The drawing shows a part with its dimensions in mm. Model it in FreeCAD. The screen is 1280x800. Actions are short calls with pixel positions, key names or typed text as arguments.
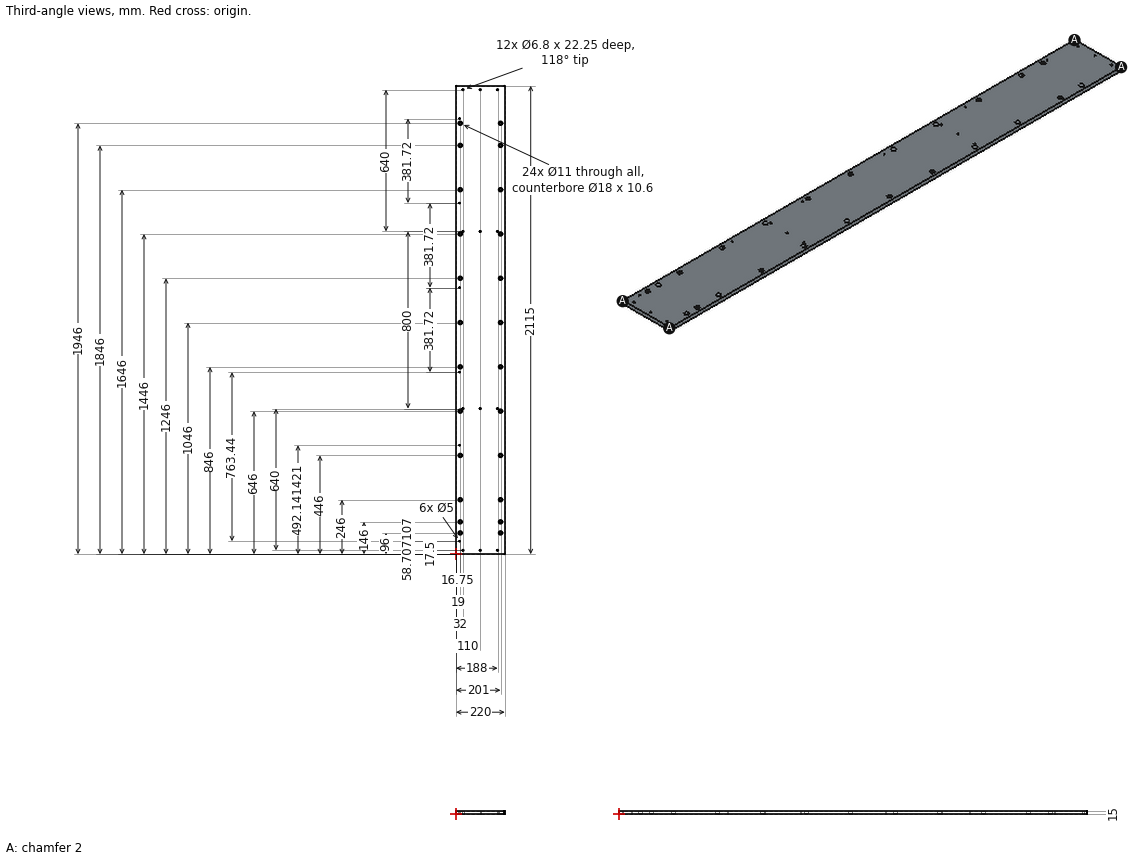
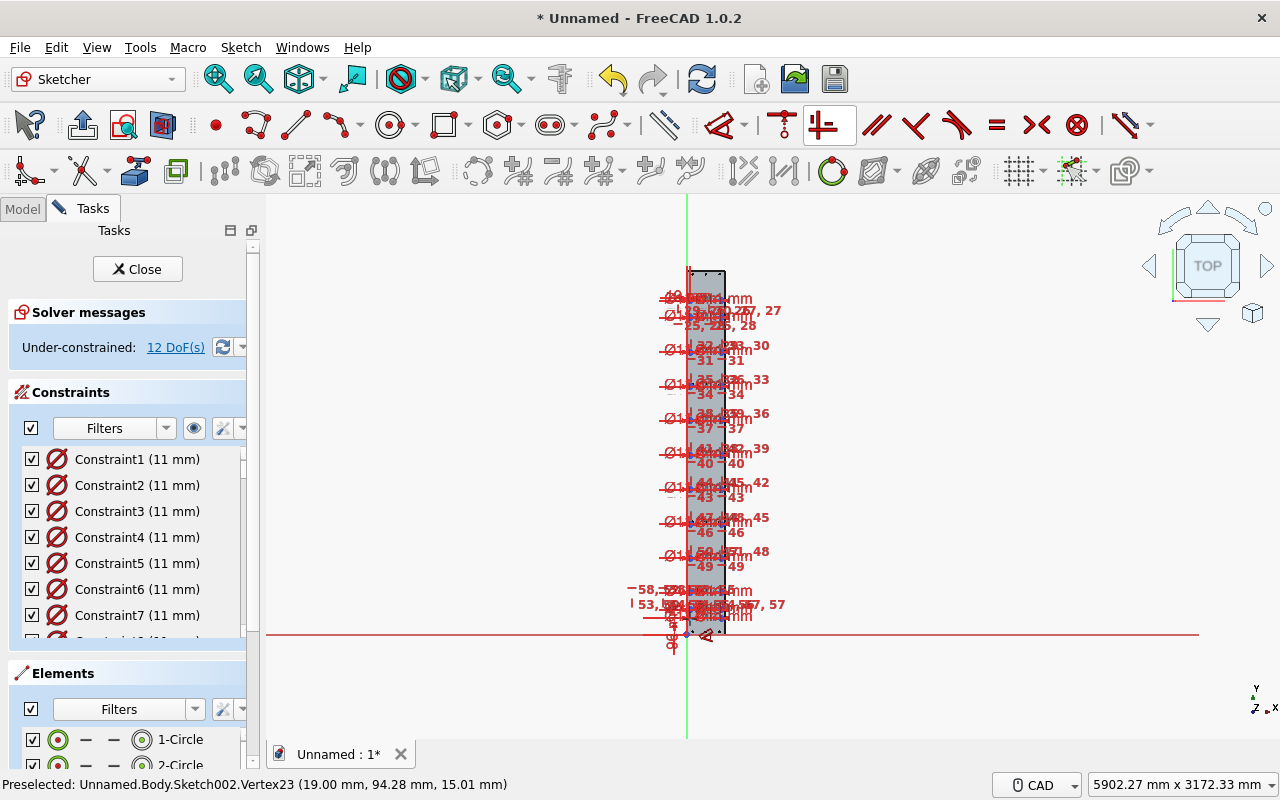
click(721, 301)
click(704, 669)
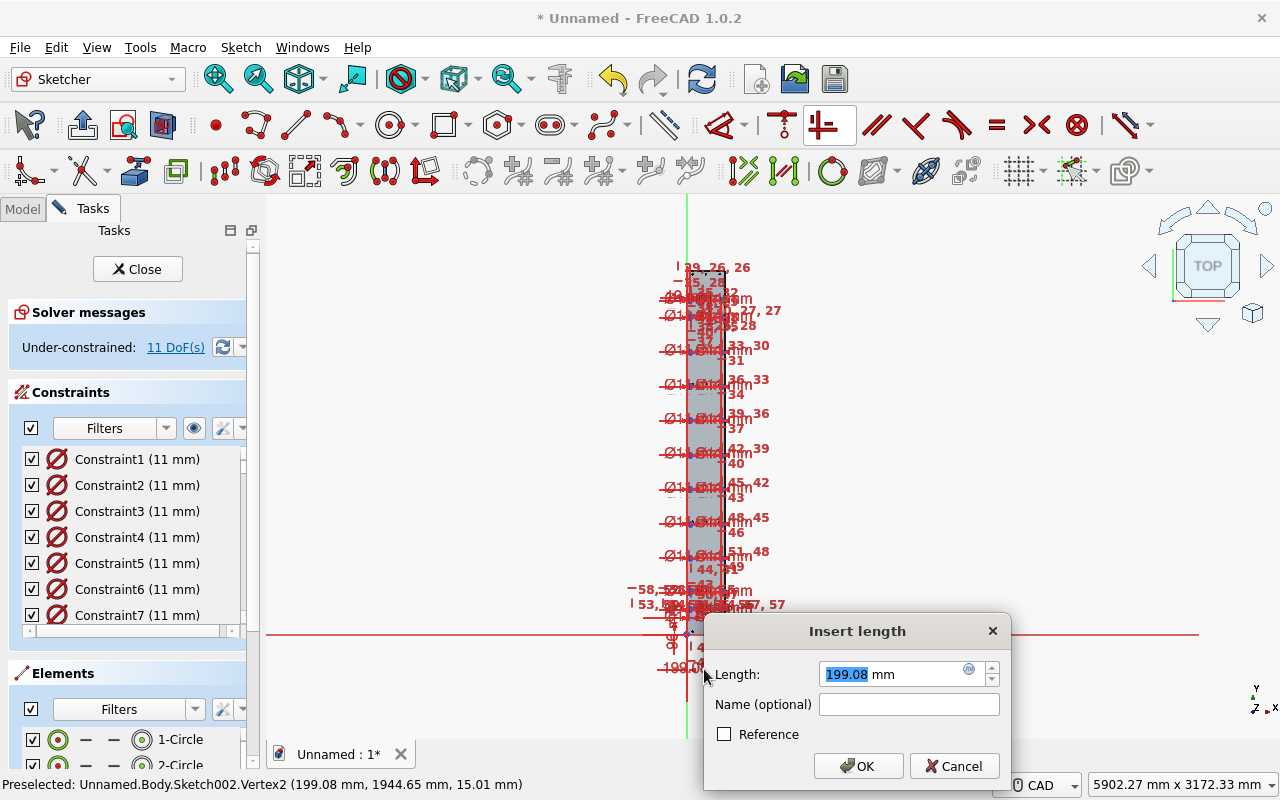
text(201)
key(Return)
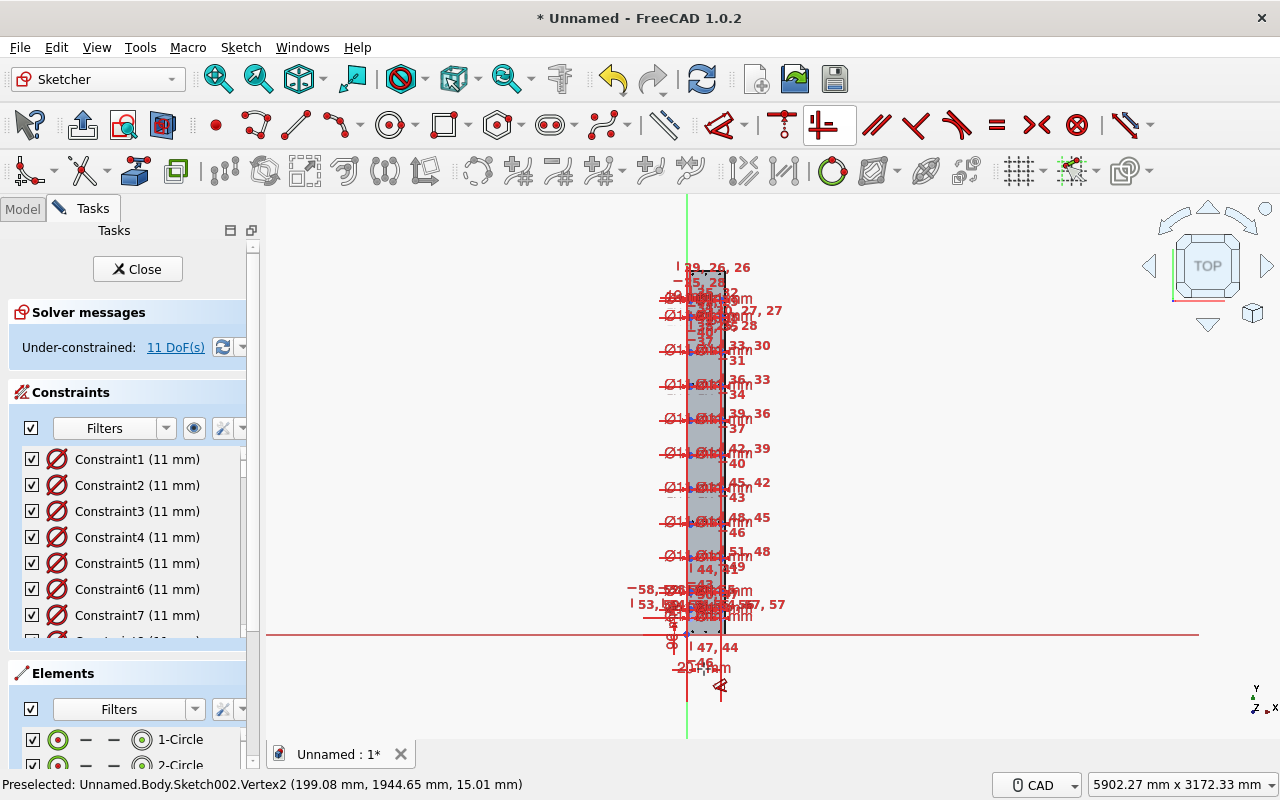
click(690, 490)
click(653, 562)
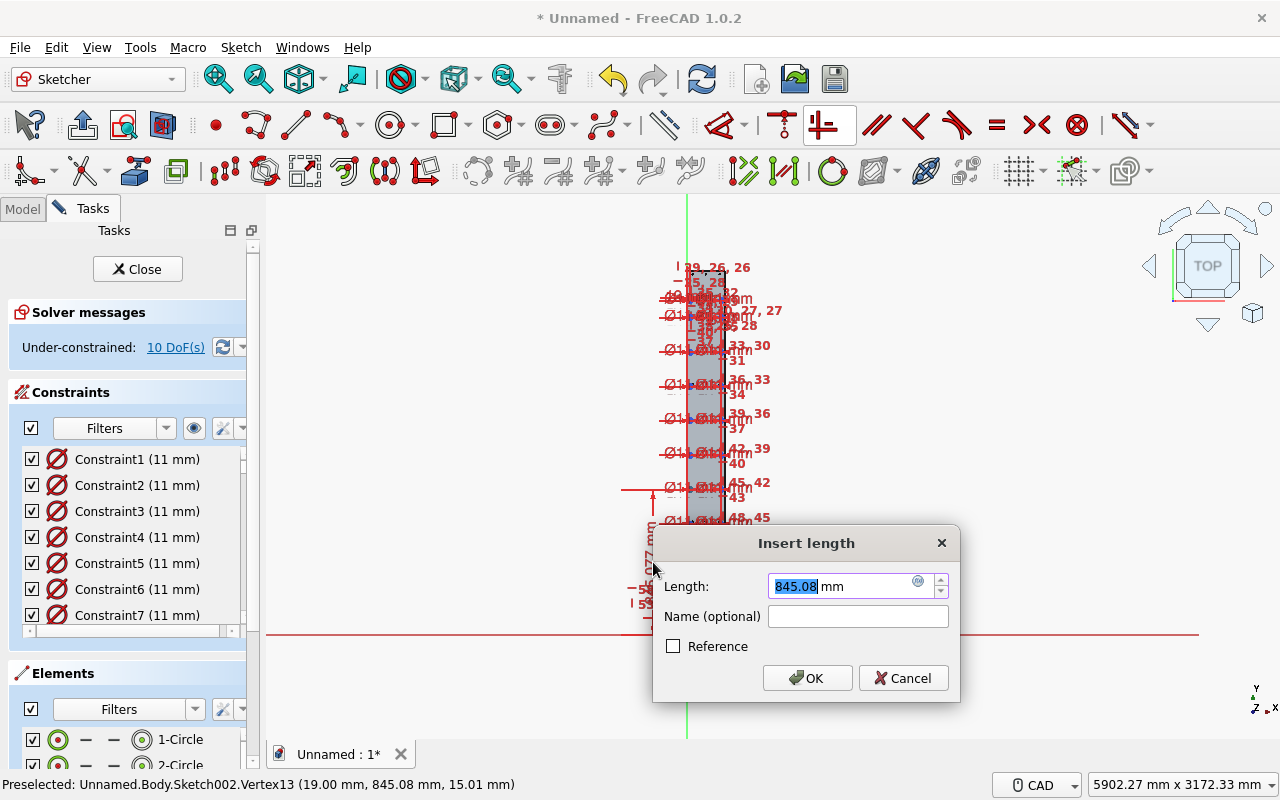
text(846)
key(Return)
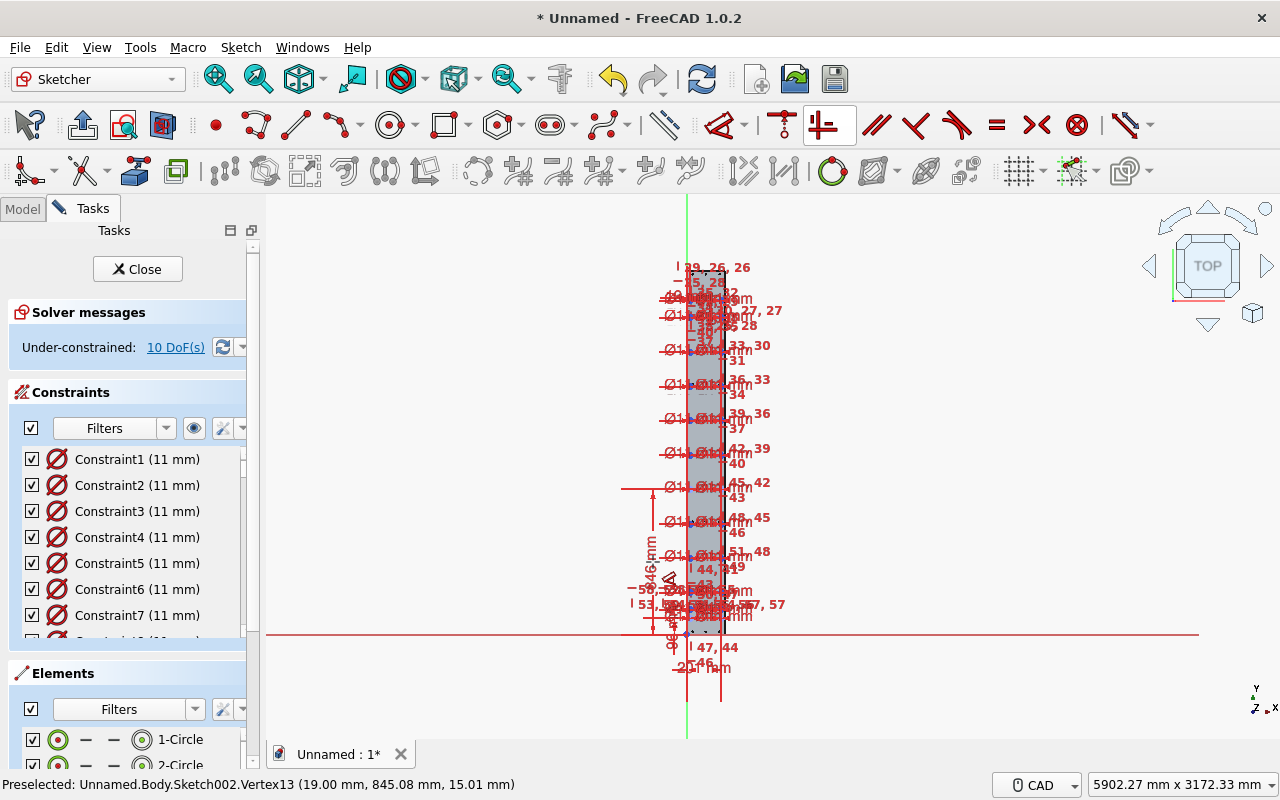
click(690, 524)
click(653, 605)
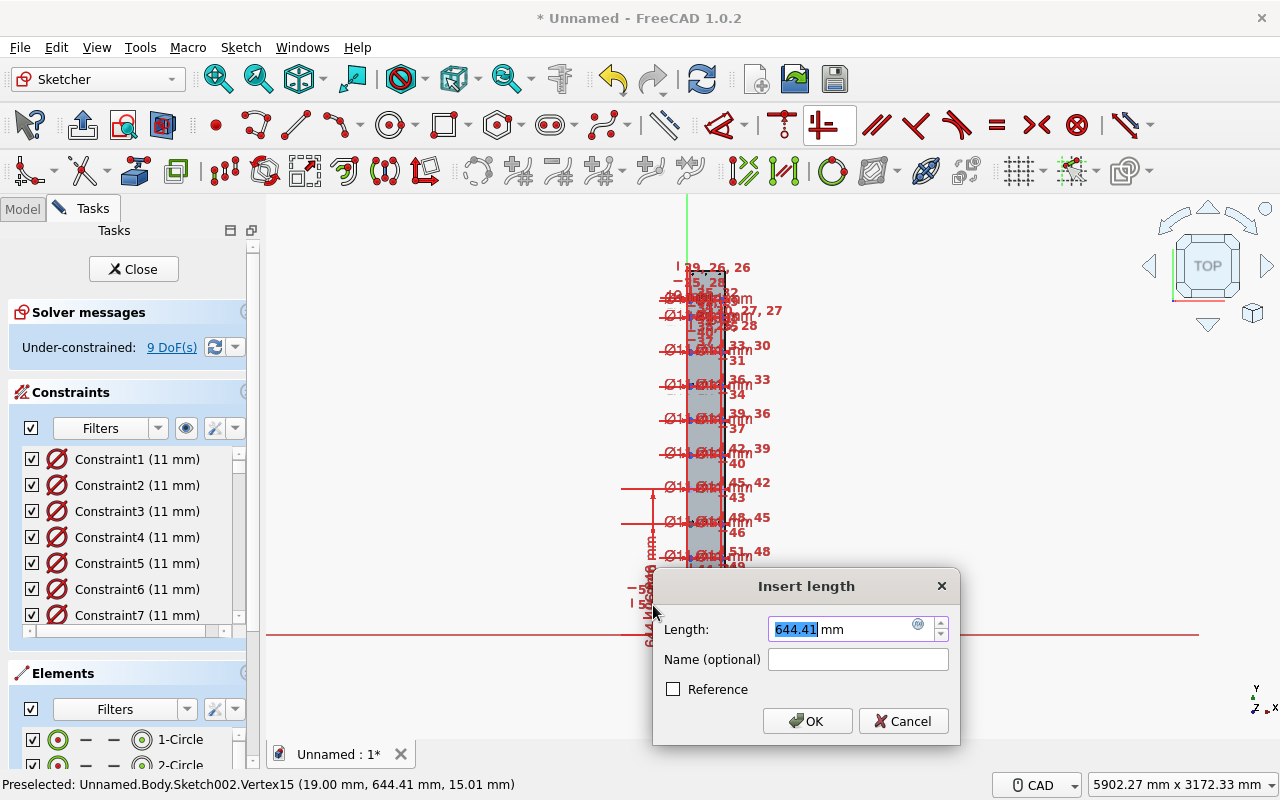
text(646)
key(Return)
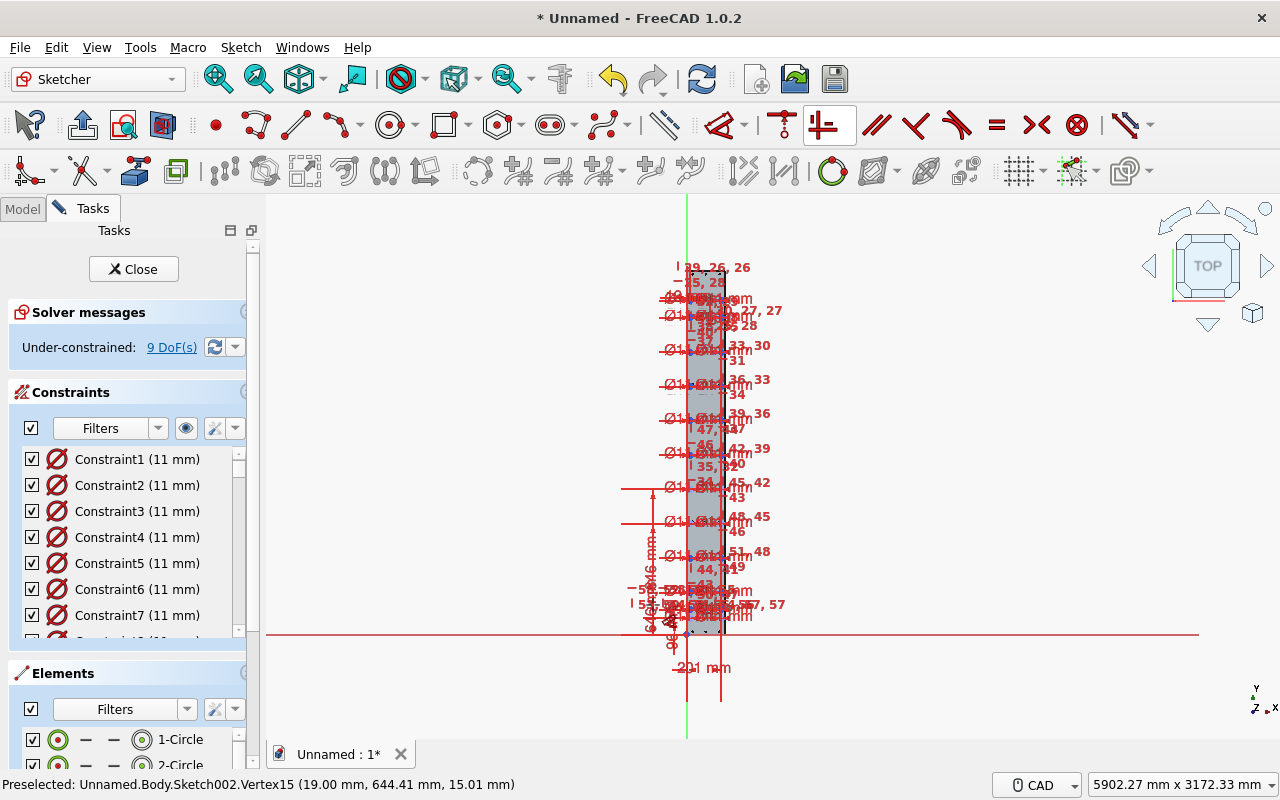
click(690, 558)
click(724, 579)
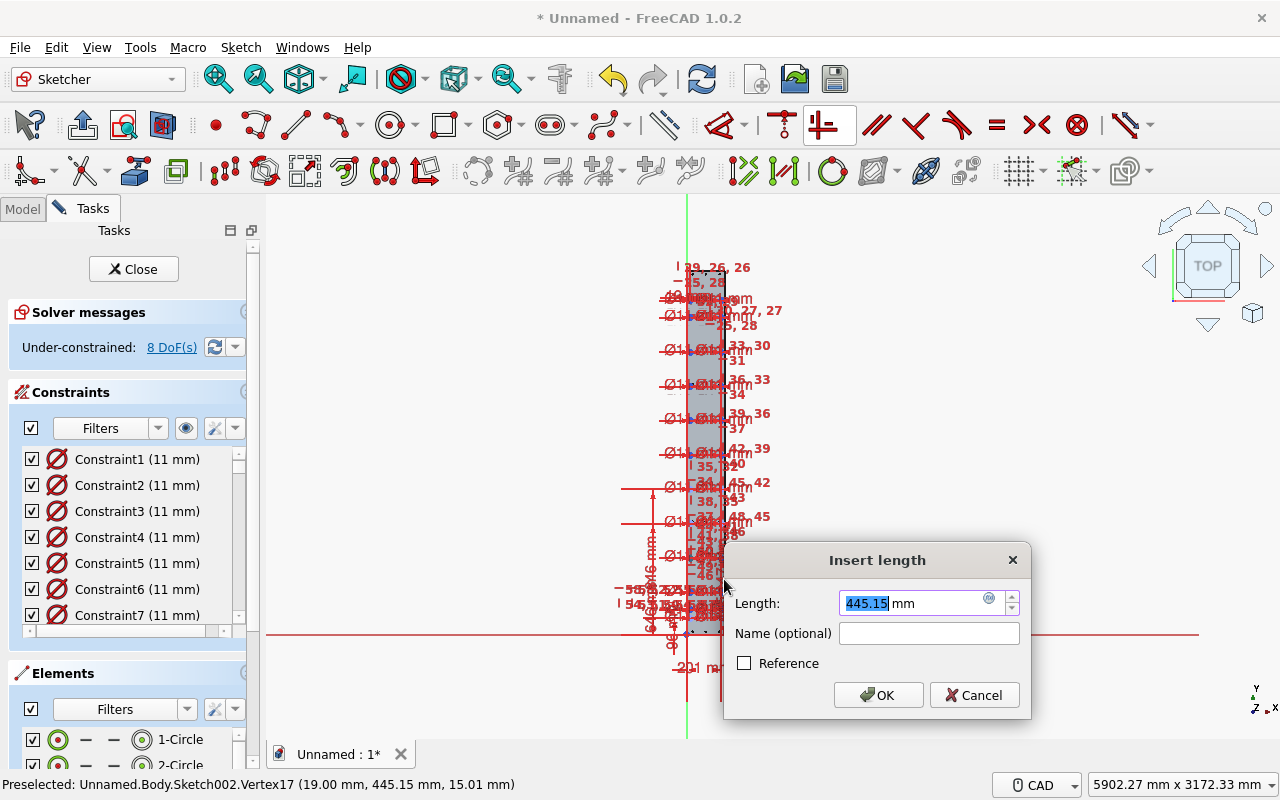
text(446)
key(Return)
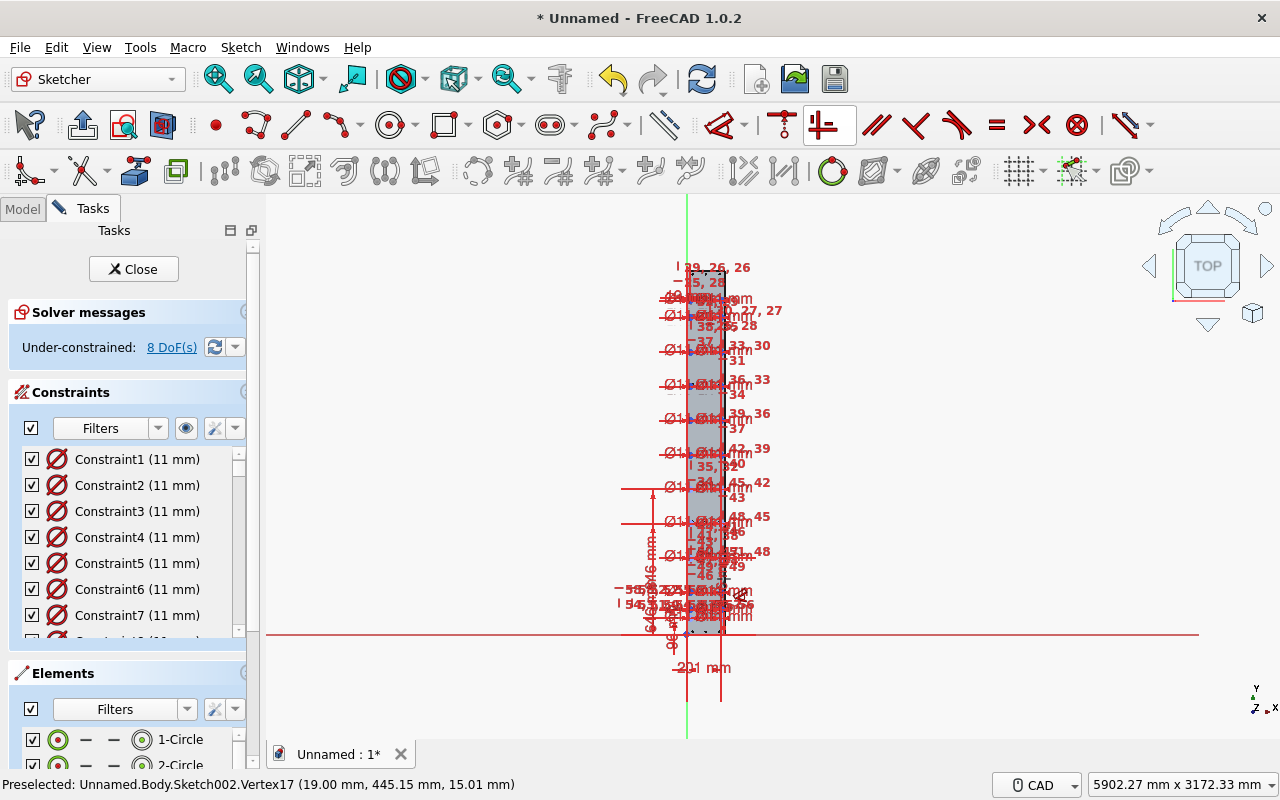
click(690, 593)
click(748, 614)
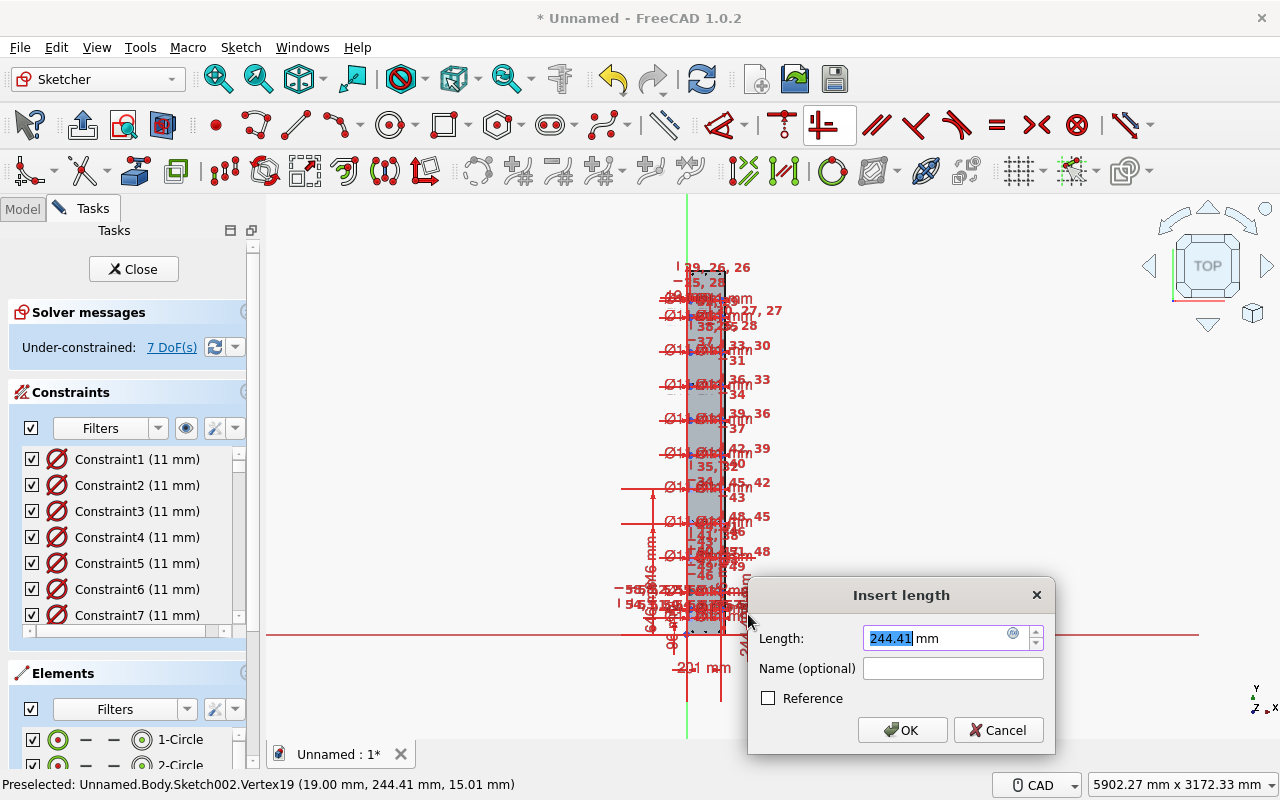
text(246)
key(Return)